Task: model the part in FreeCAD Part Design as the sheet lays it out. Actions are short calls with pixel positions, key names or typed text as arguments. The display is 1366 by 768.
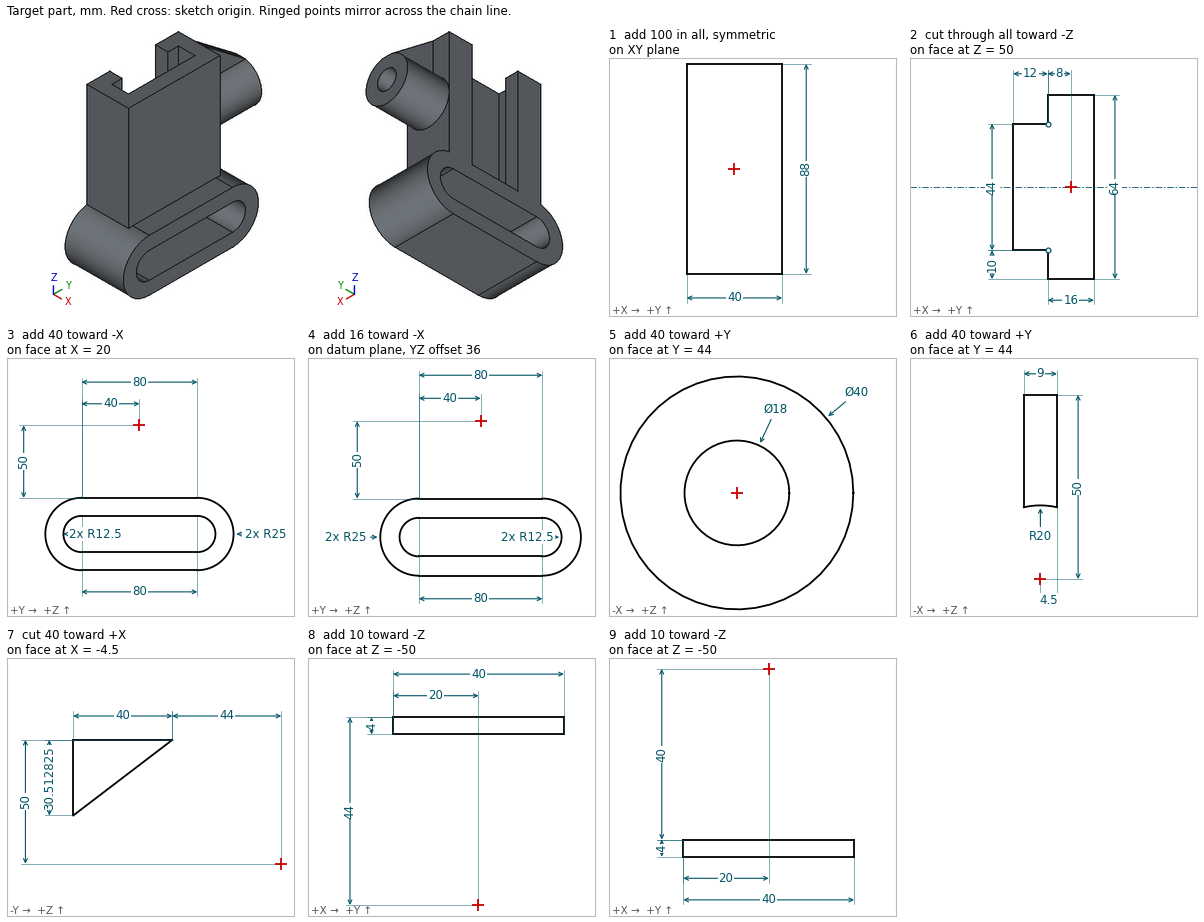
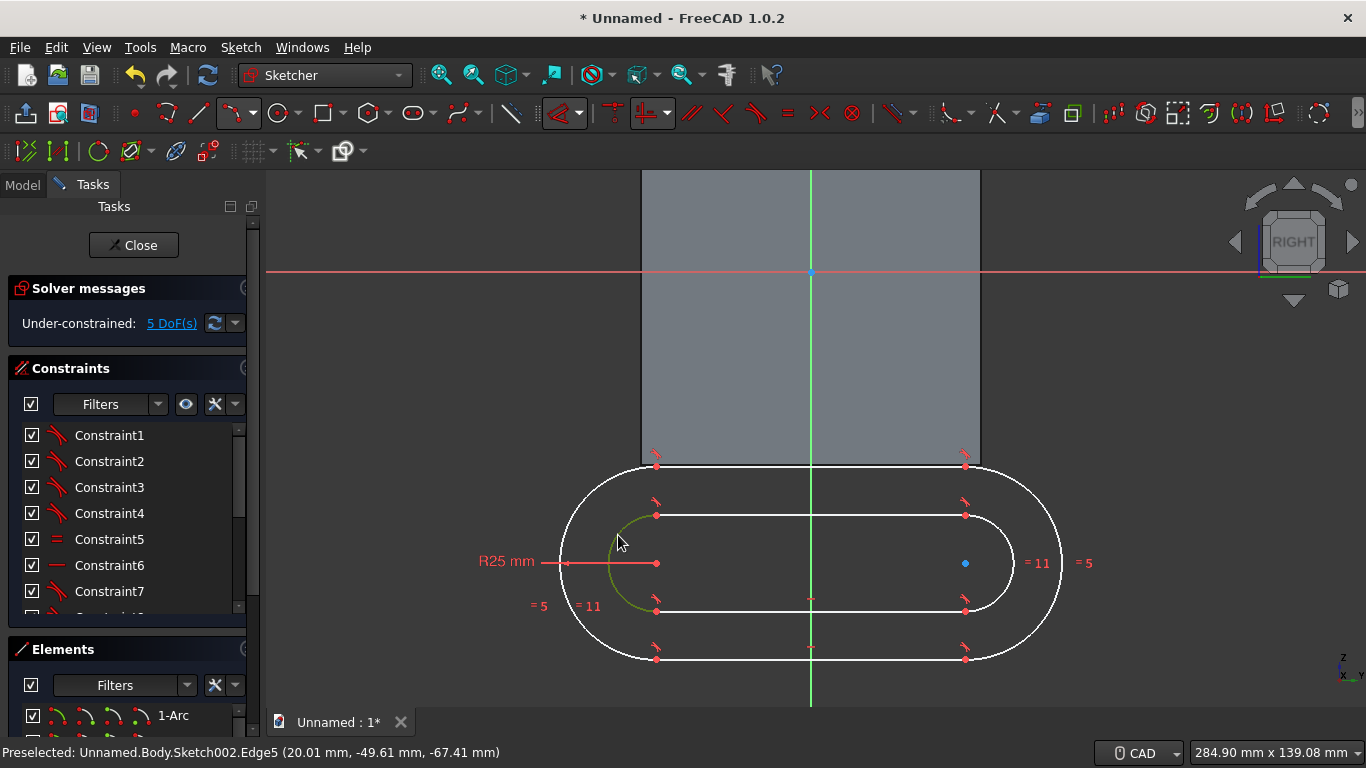
key(k)
key(r)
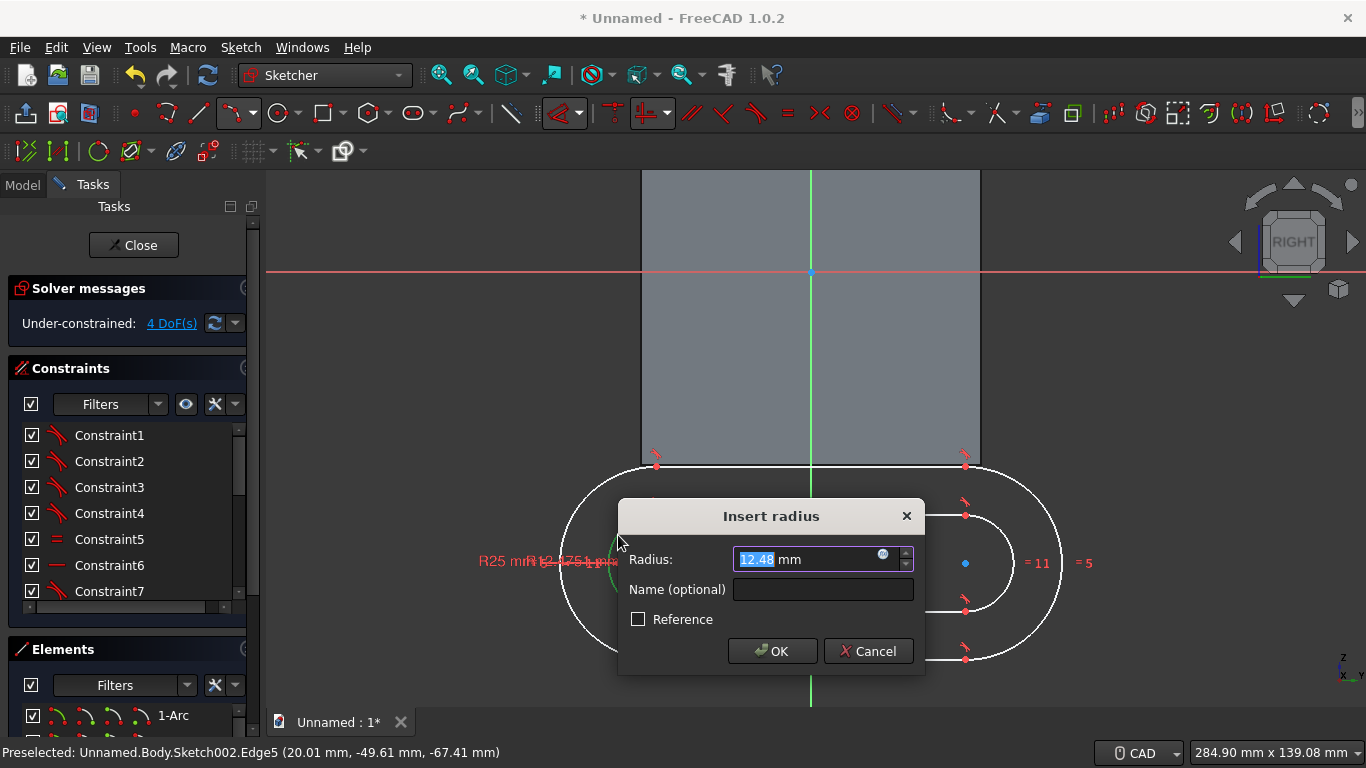
text(12.5)
key(Return)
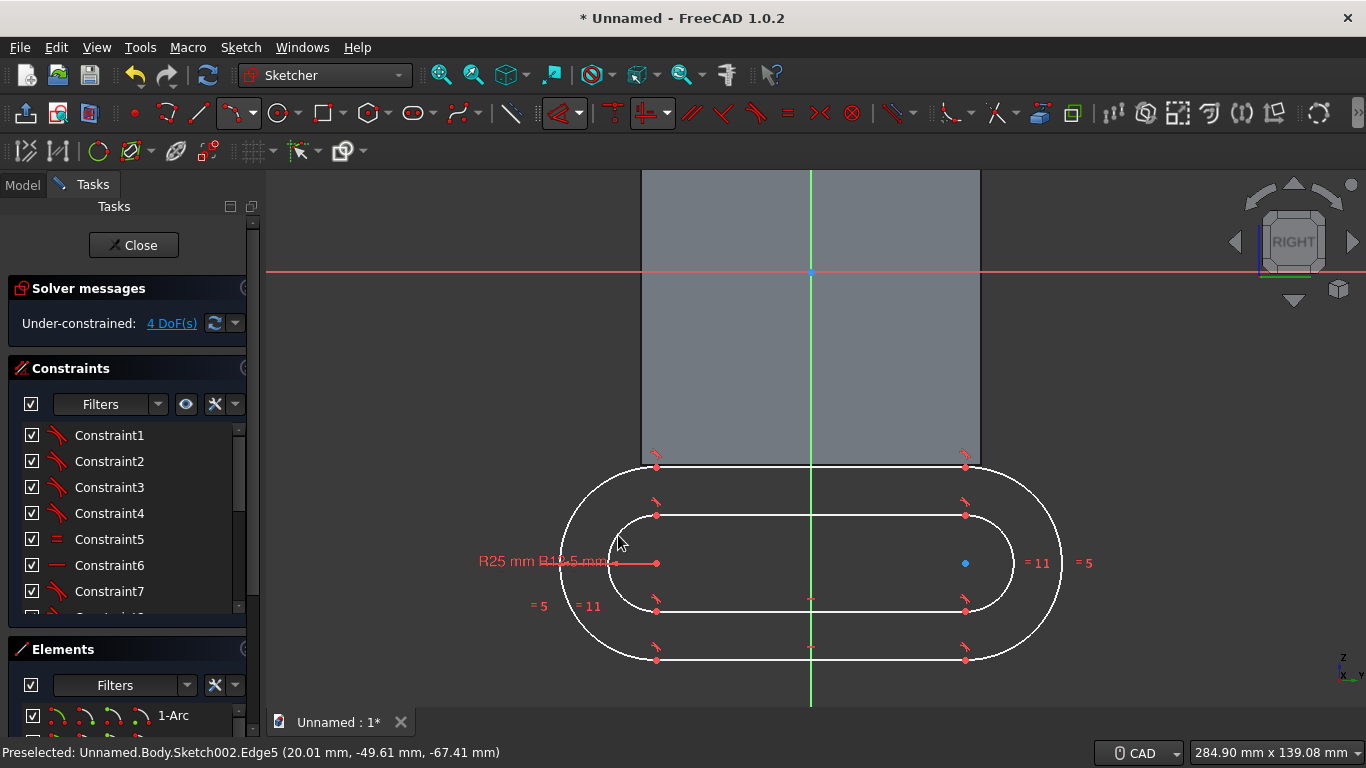
click(749, 467)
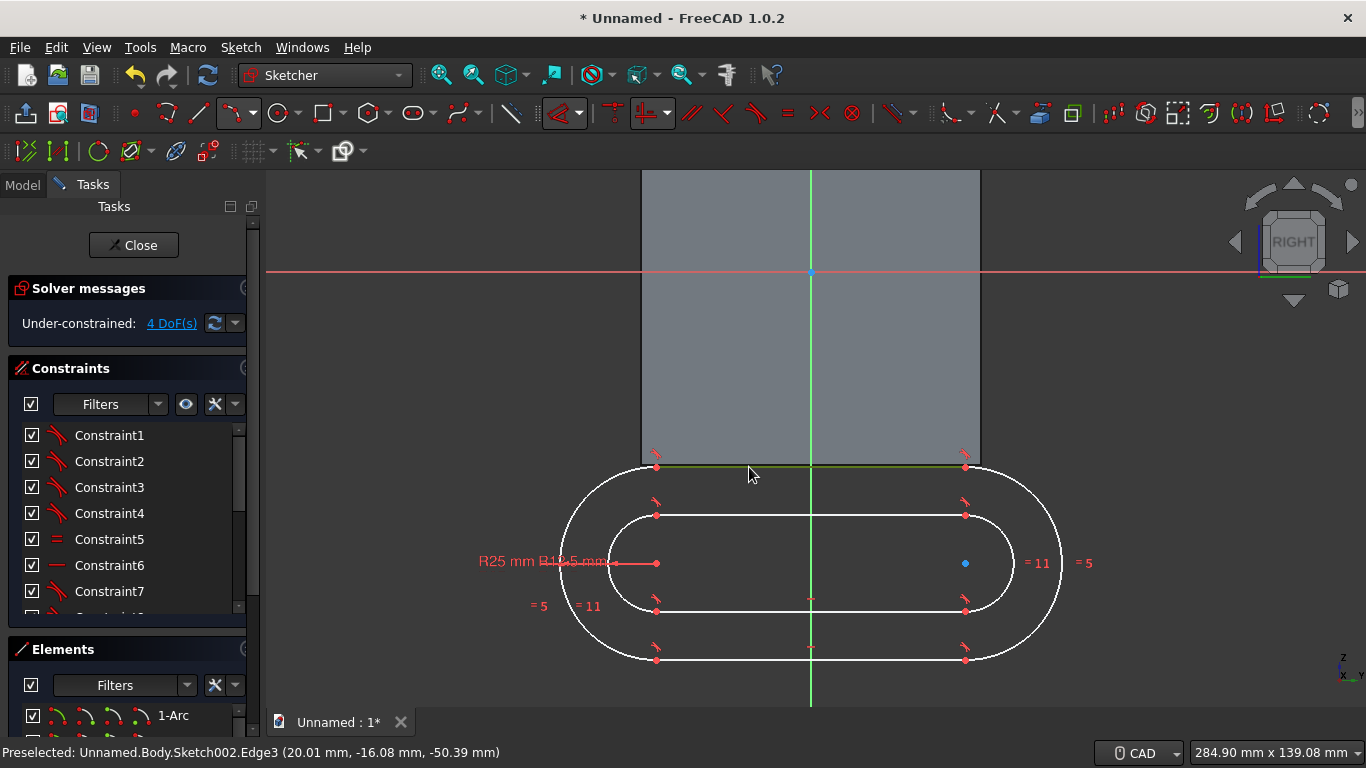
key(l)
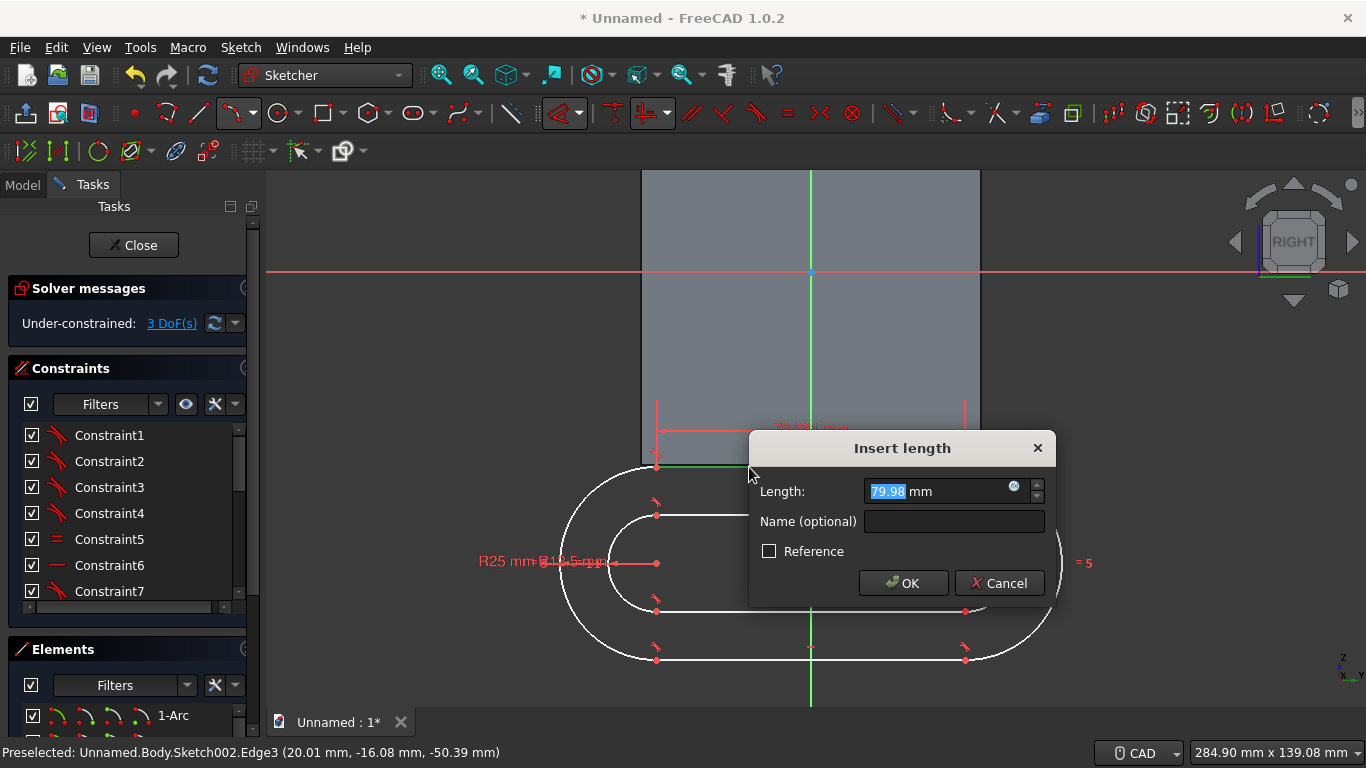
text(80)
key(Return)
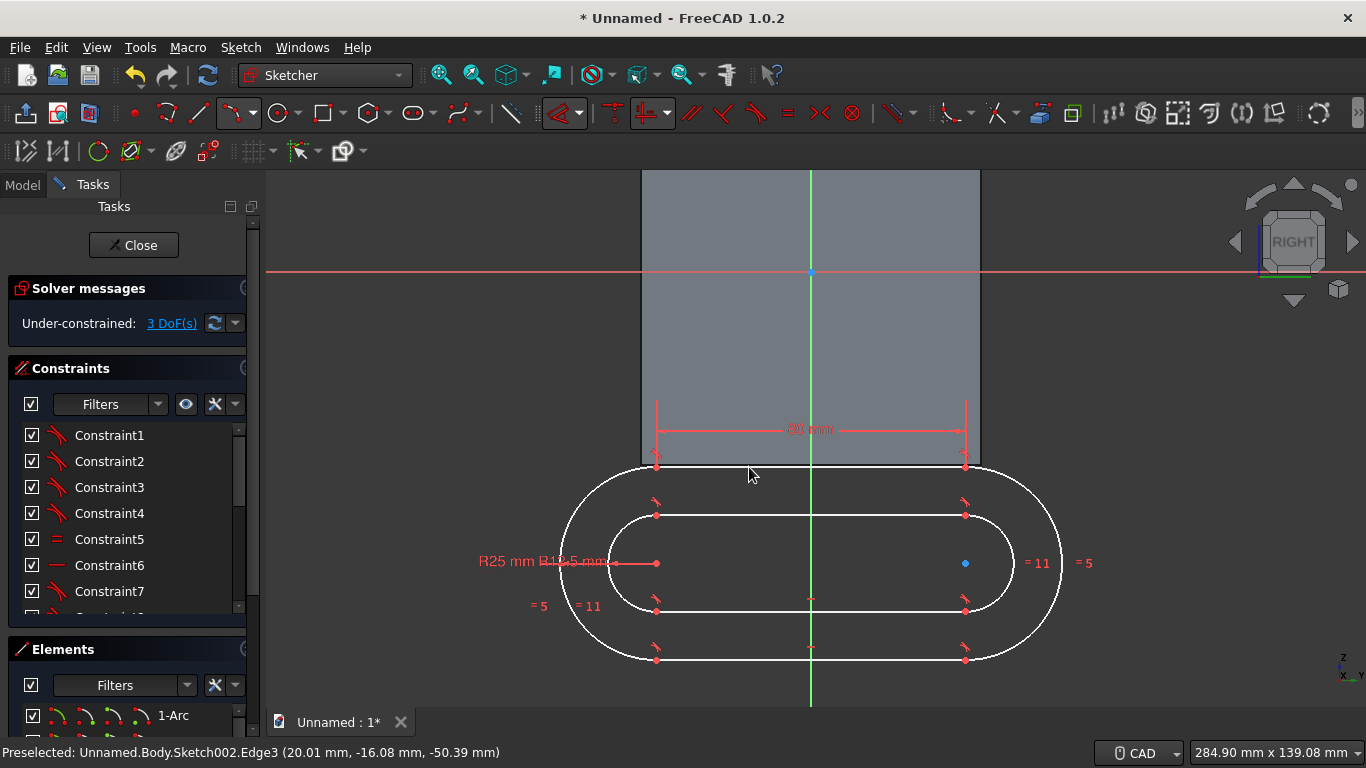
click(749, 515)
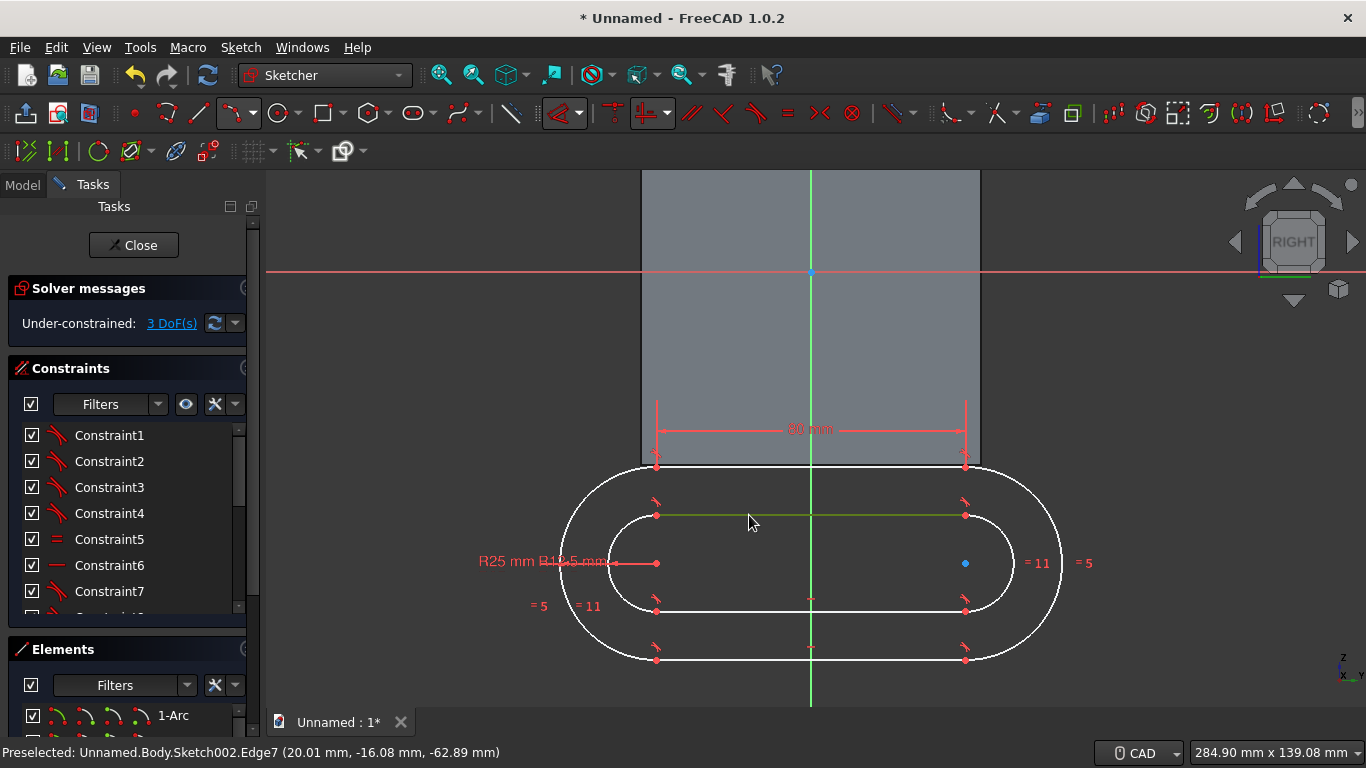
key(l)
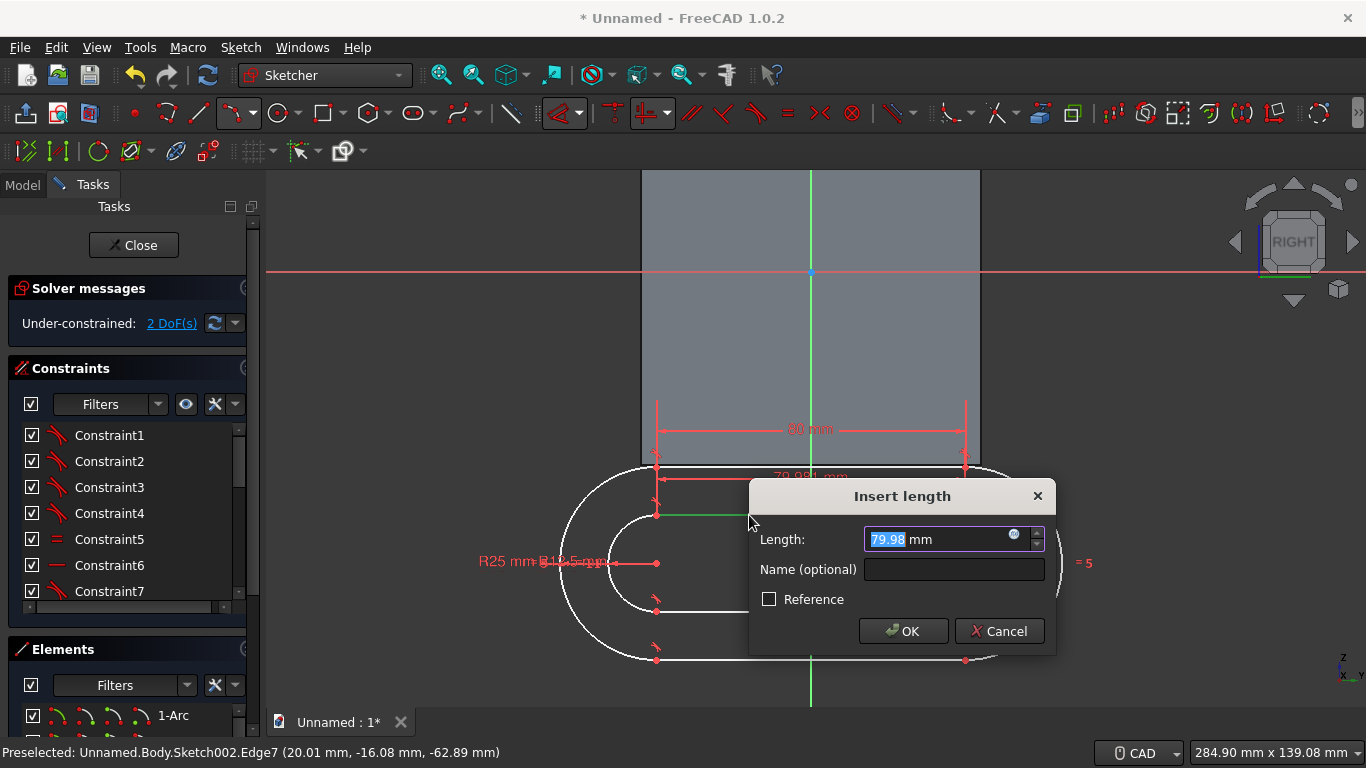
text(80)
key(Return)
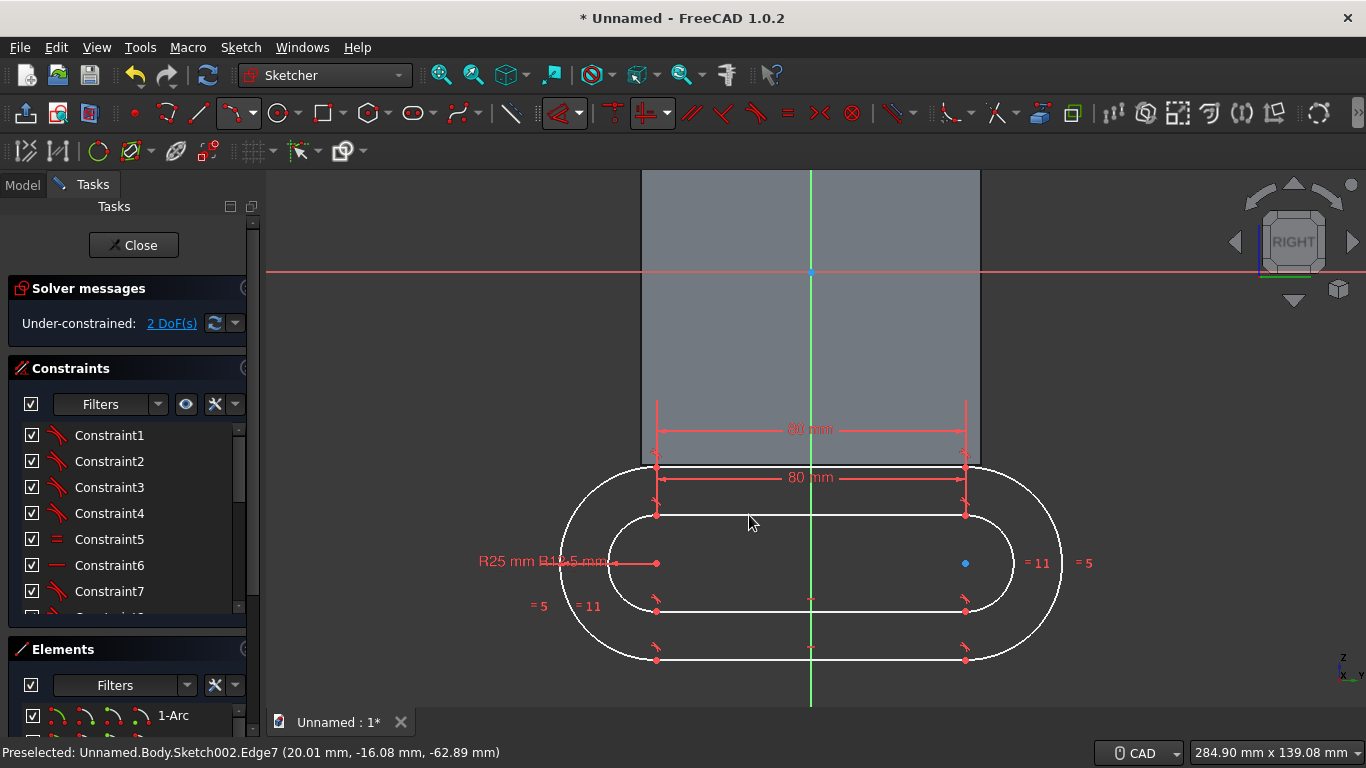
click(657, 467)